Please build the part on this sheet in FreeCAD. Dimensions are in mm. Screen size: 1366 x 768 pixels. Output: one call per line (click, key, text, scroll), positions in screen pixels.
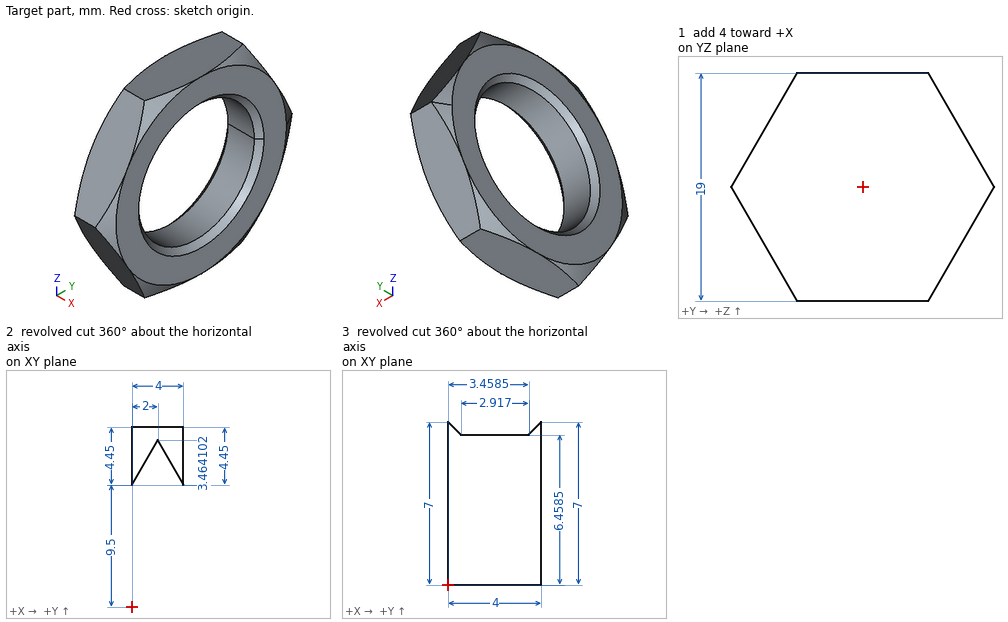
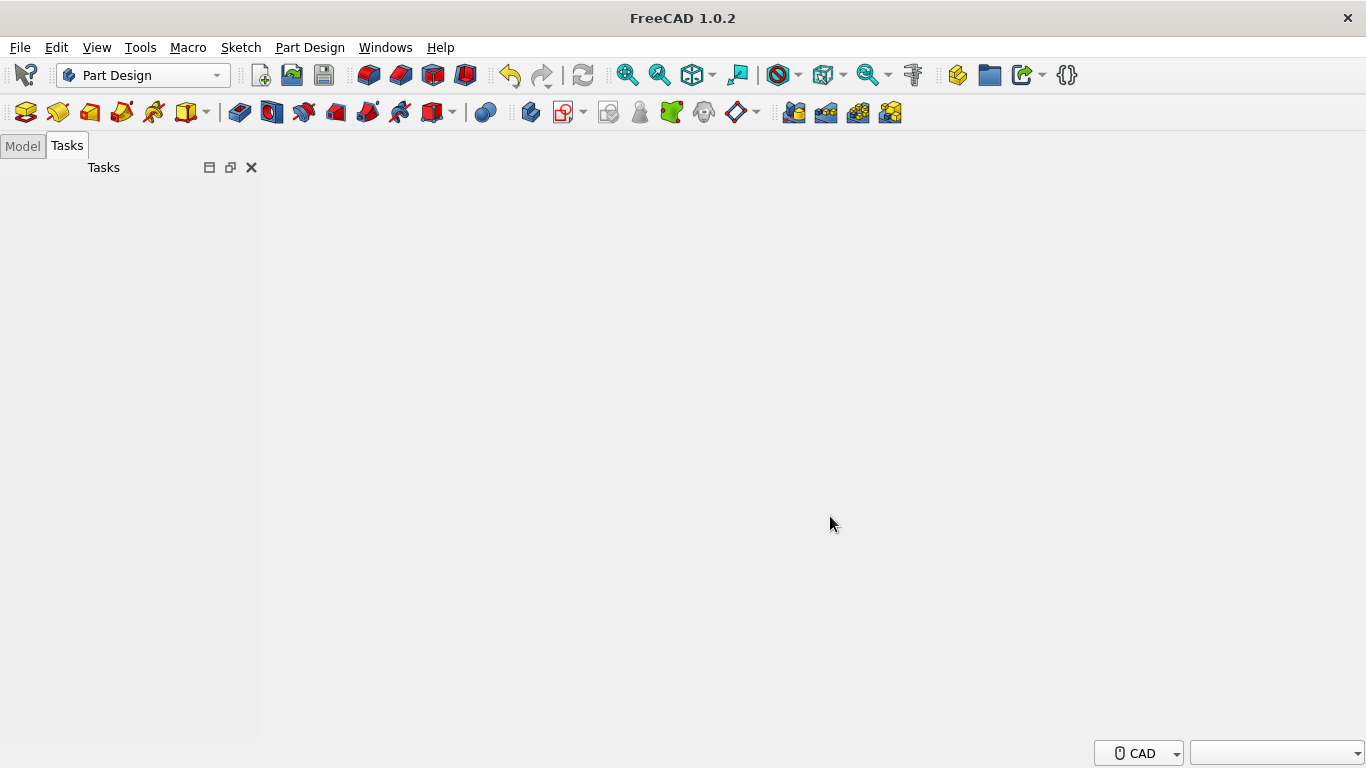
key(ctrl+n)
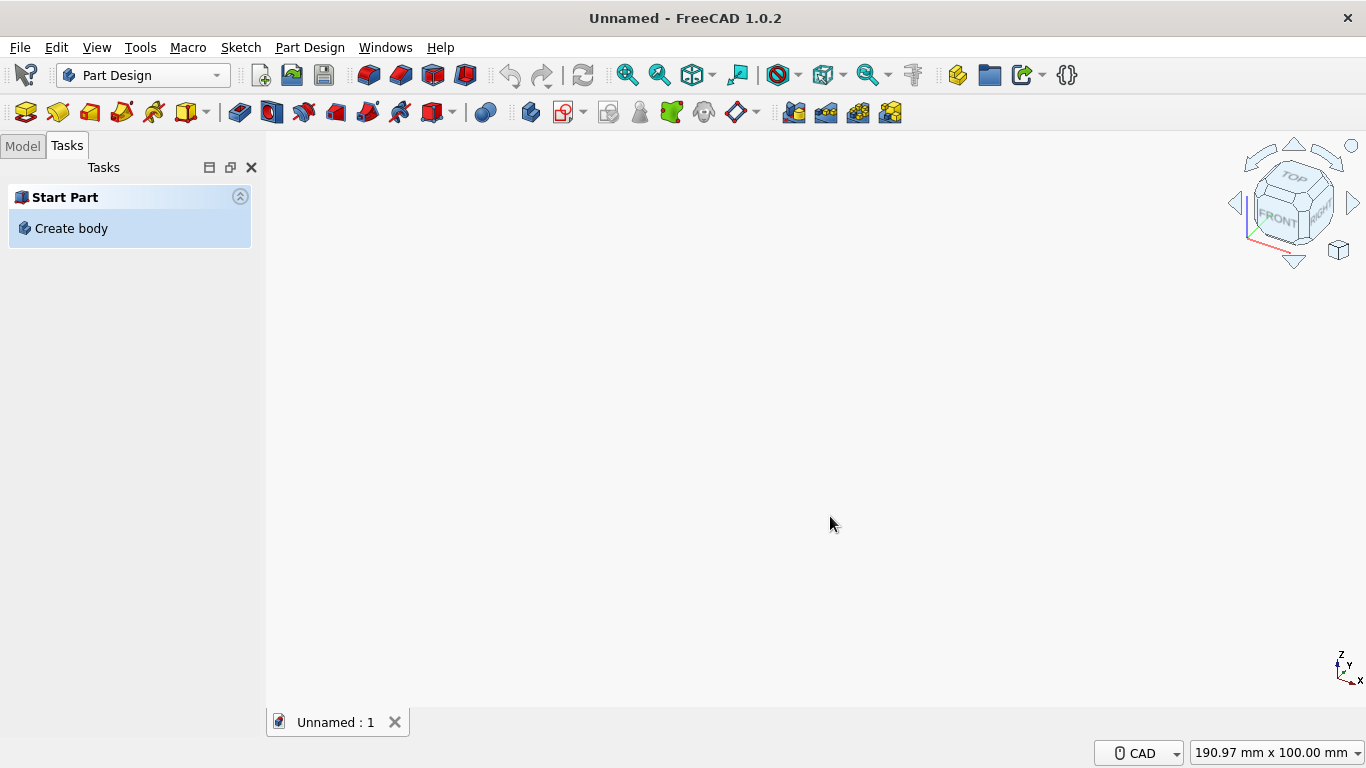
click(564, 112)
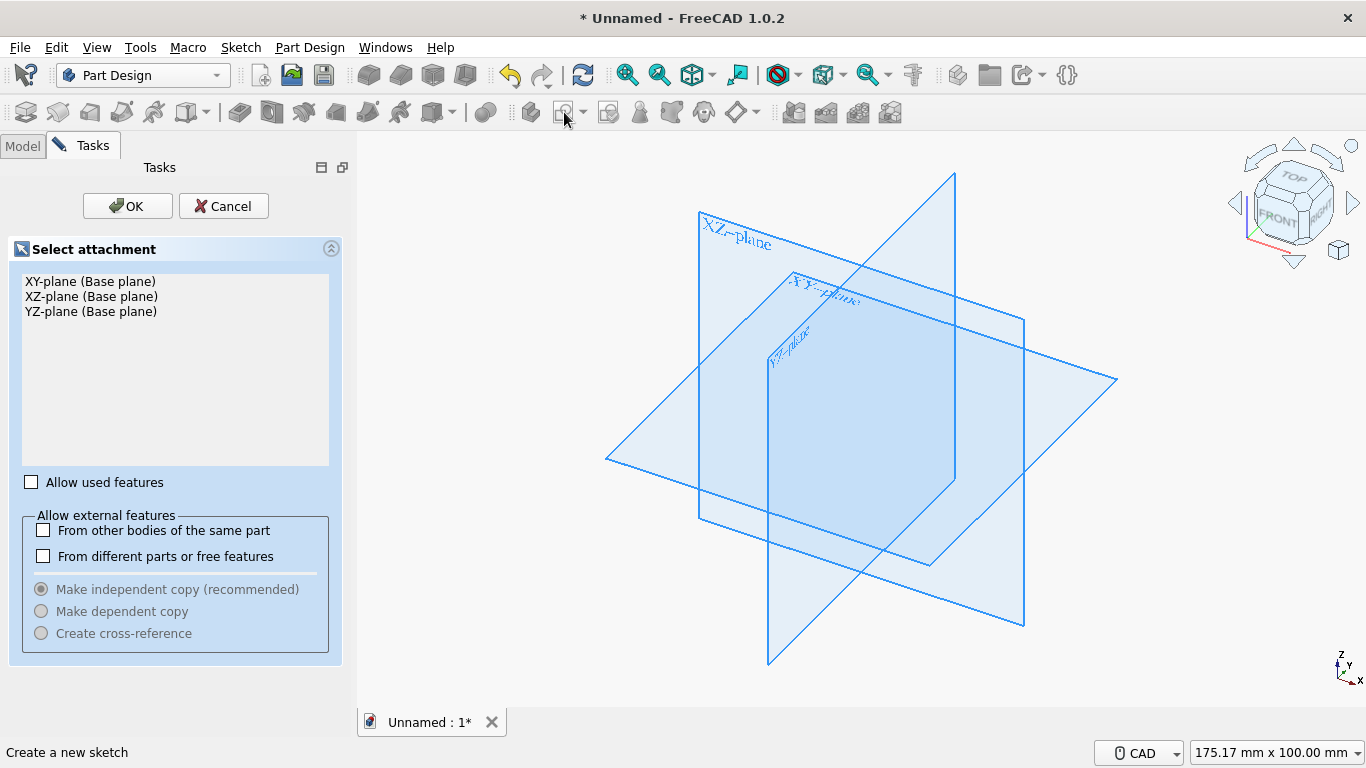
click(82, 312)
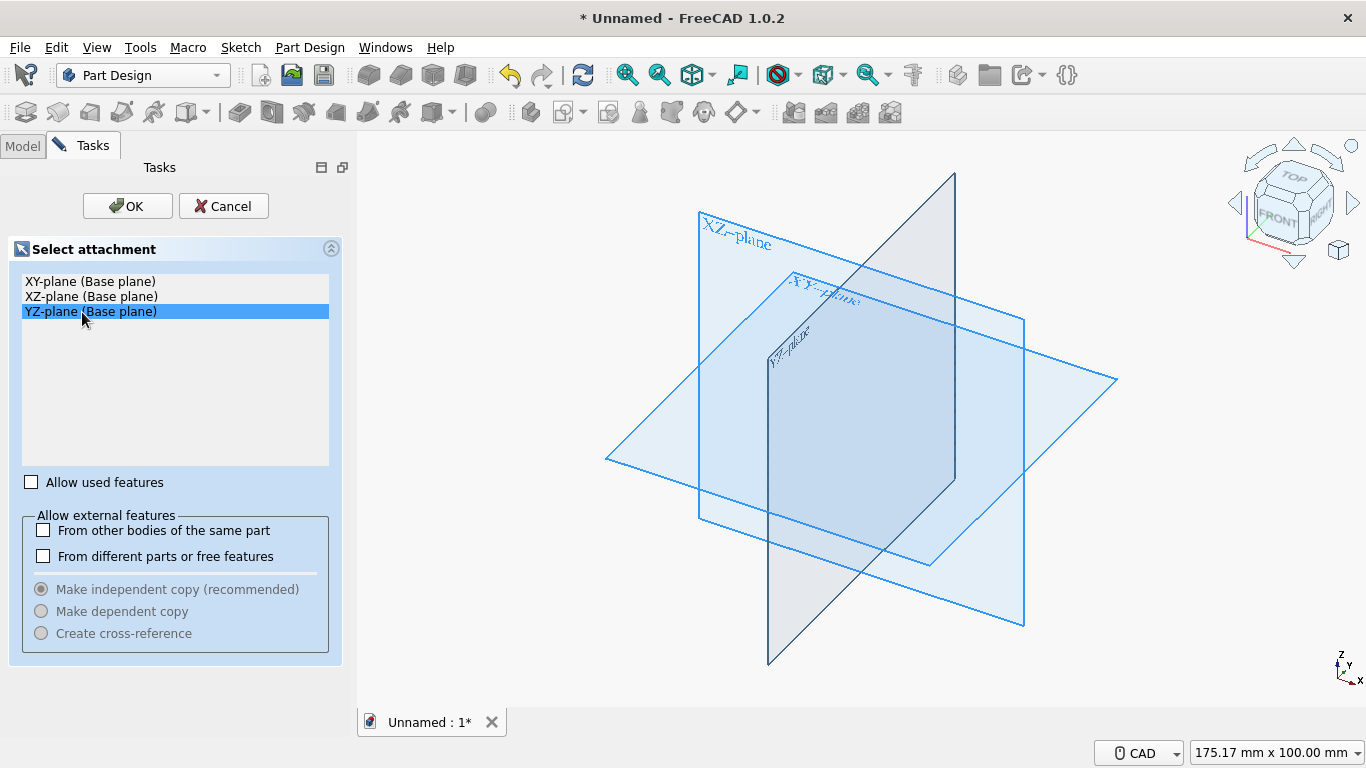
click(128, 206)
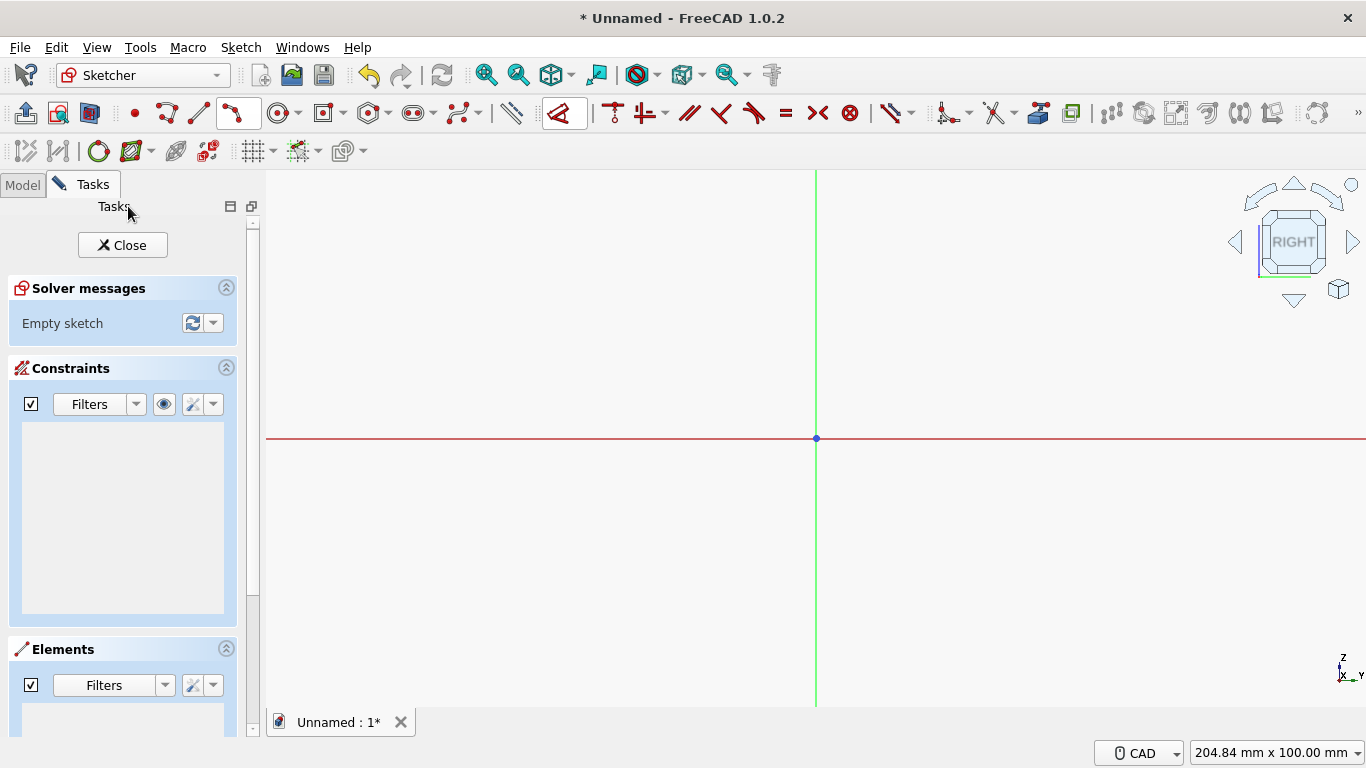
scroll(846, 438, up, 6)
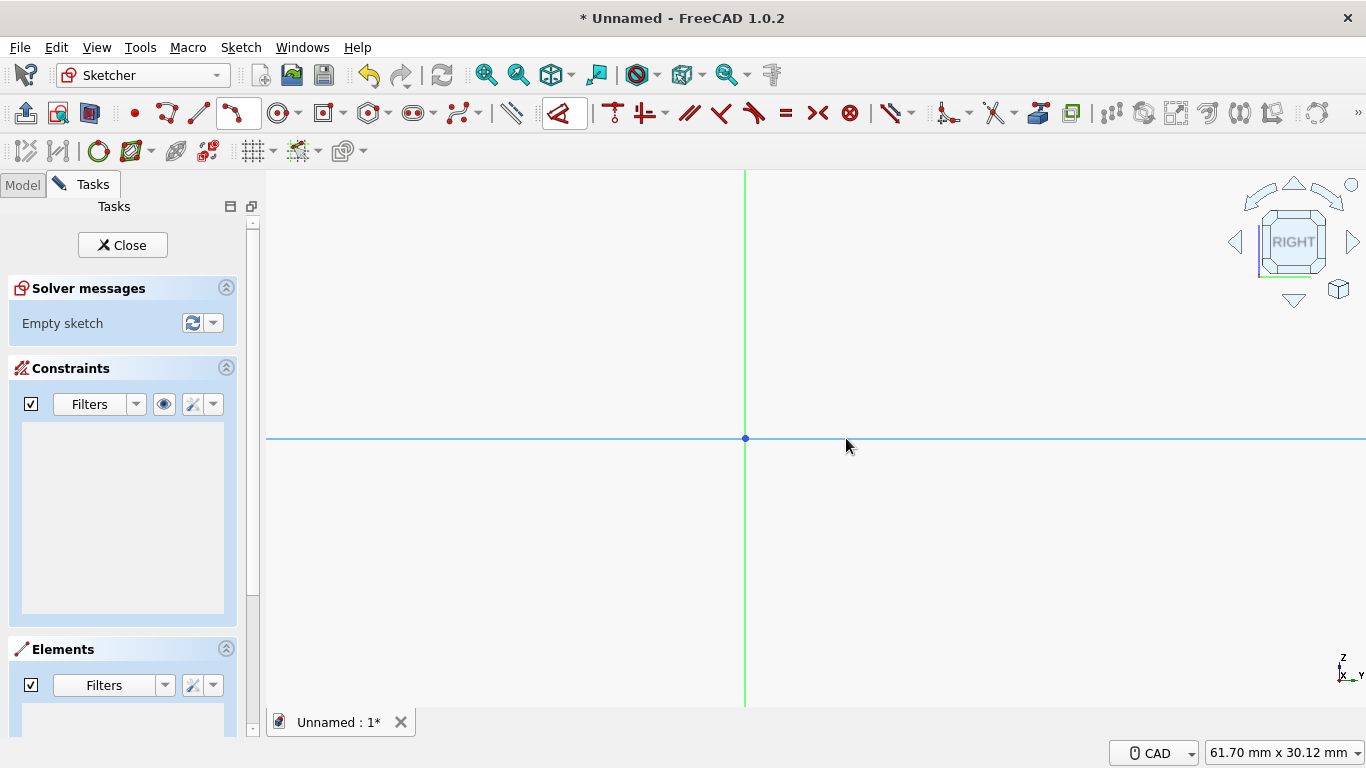
key(g)
key(p)
key(6)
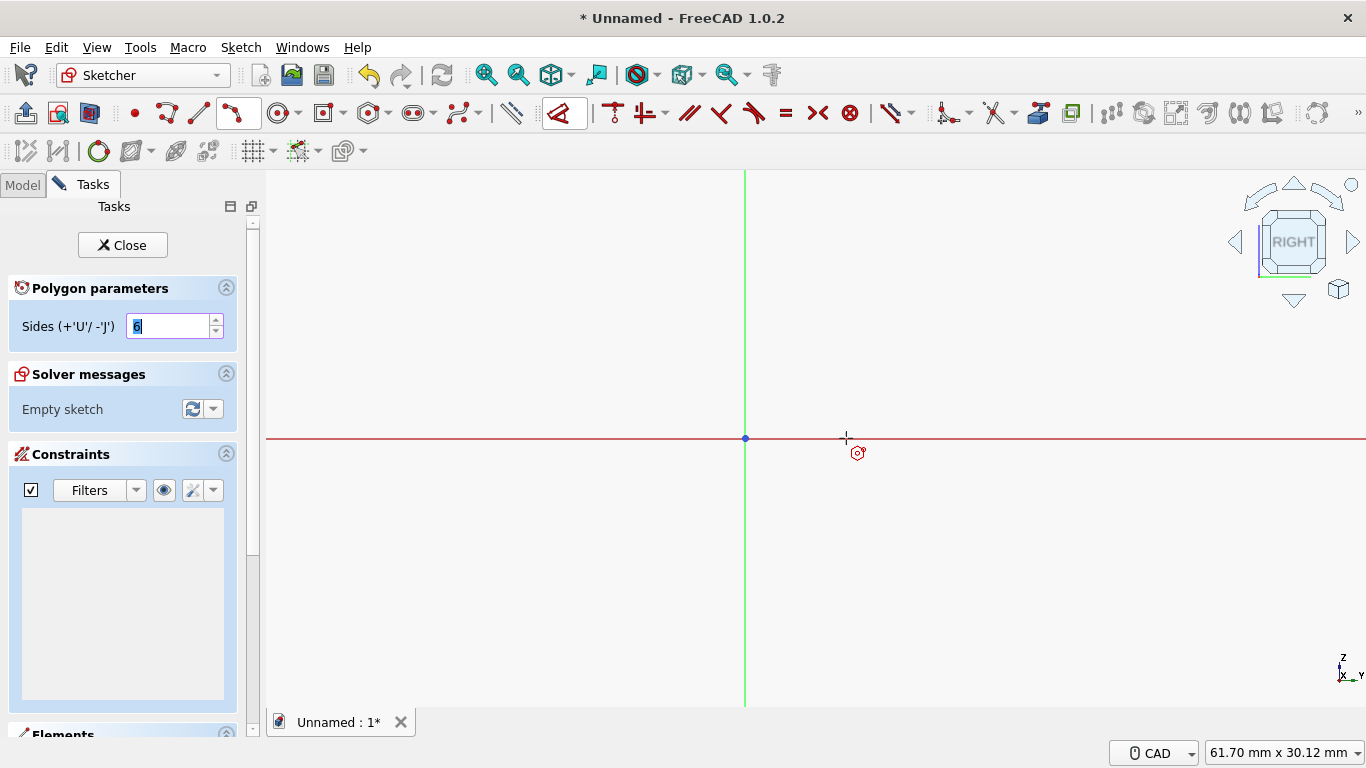
click(745, 438)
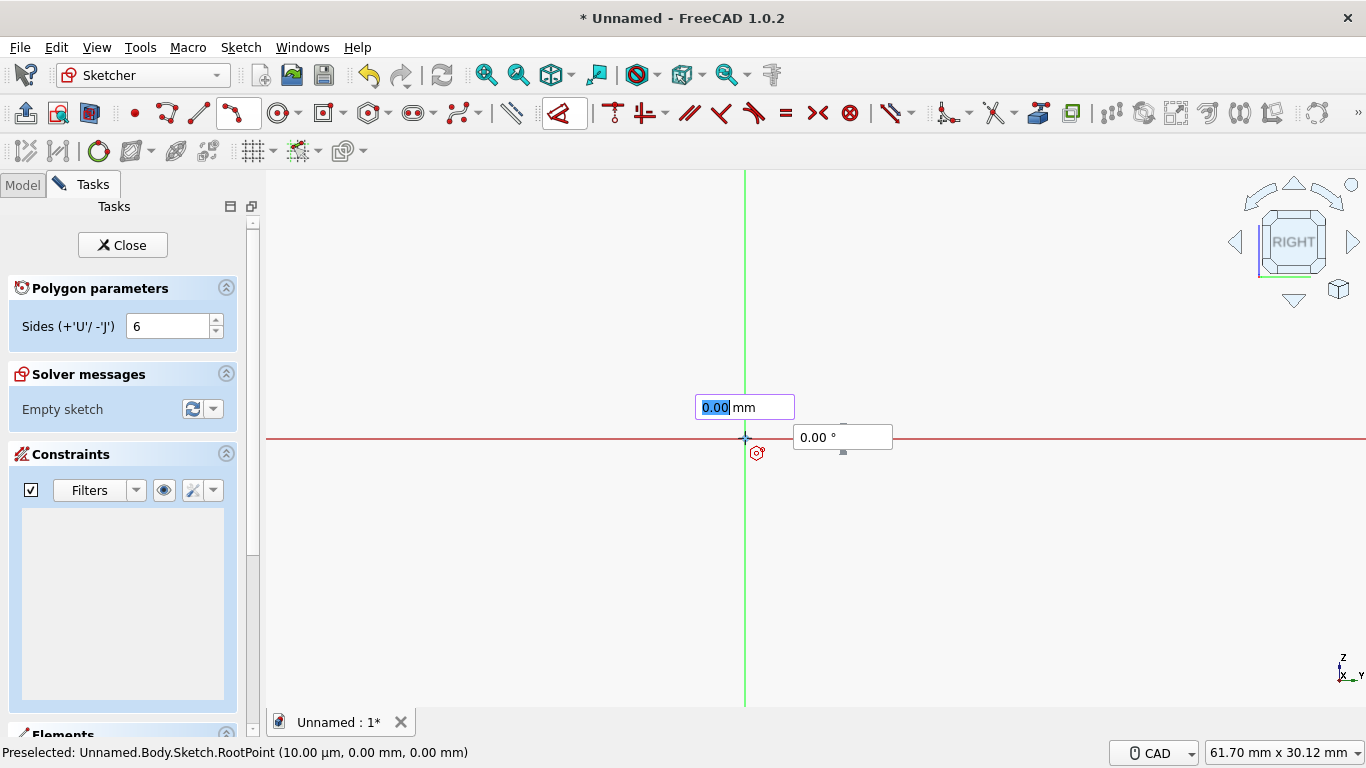
click(550, 438)
right_click(550, 438)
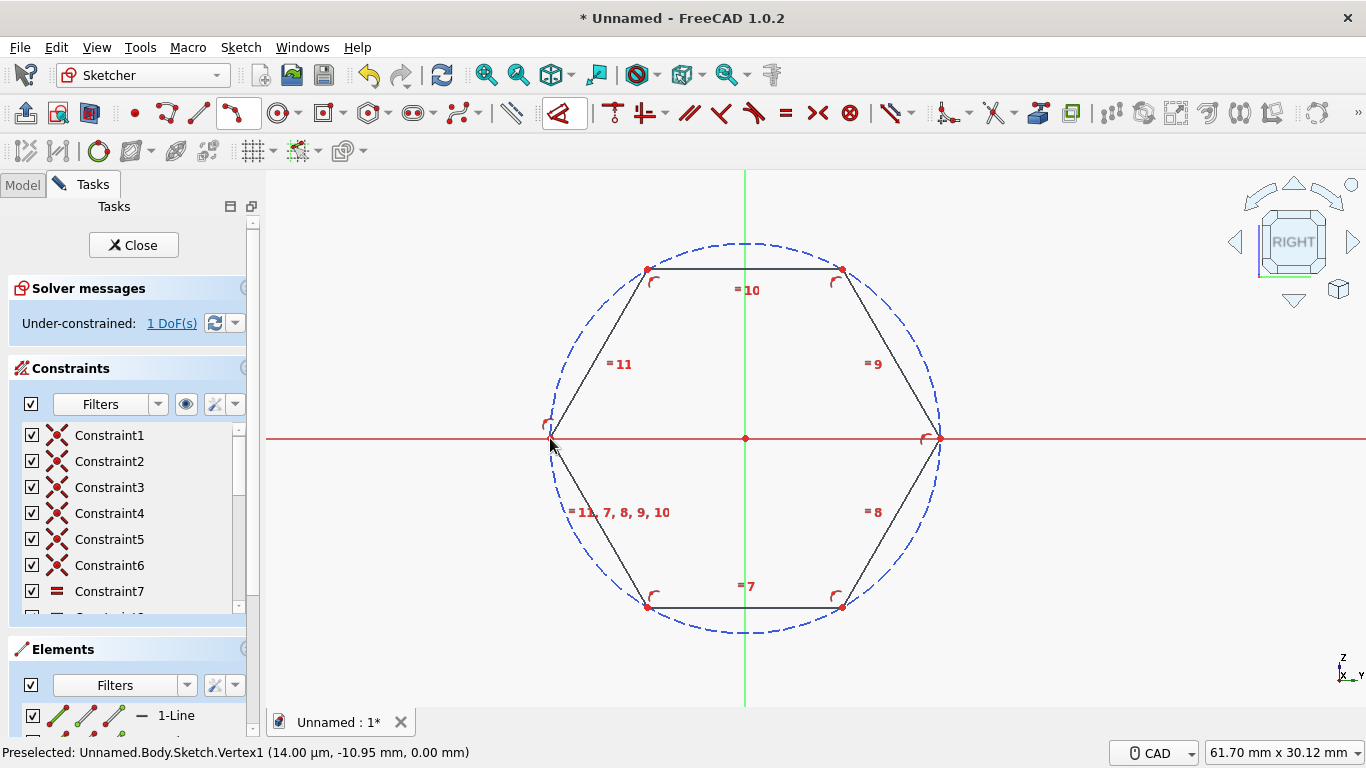
click(648, 608)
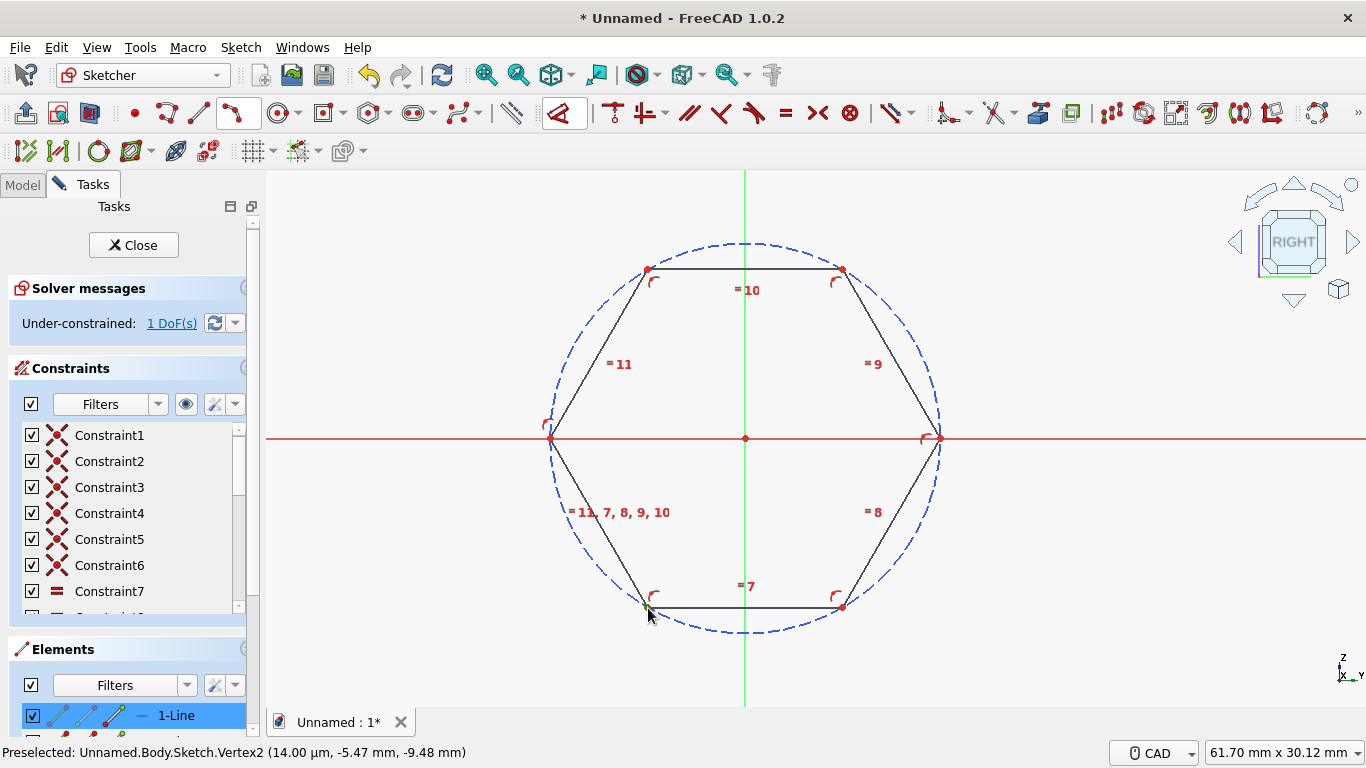
click(843, 269)